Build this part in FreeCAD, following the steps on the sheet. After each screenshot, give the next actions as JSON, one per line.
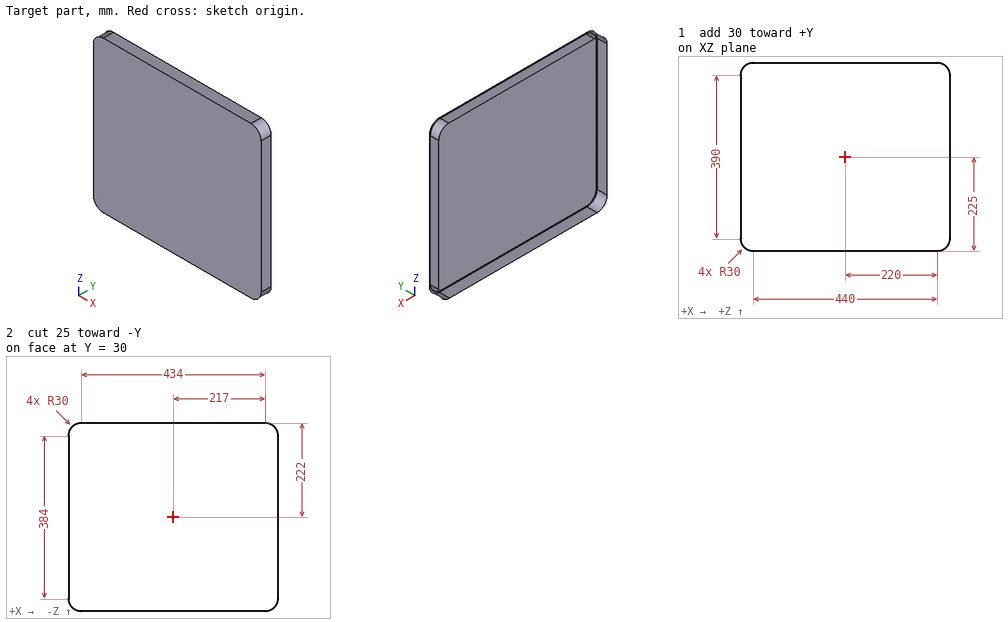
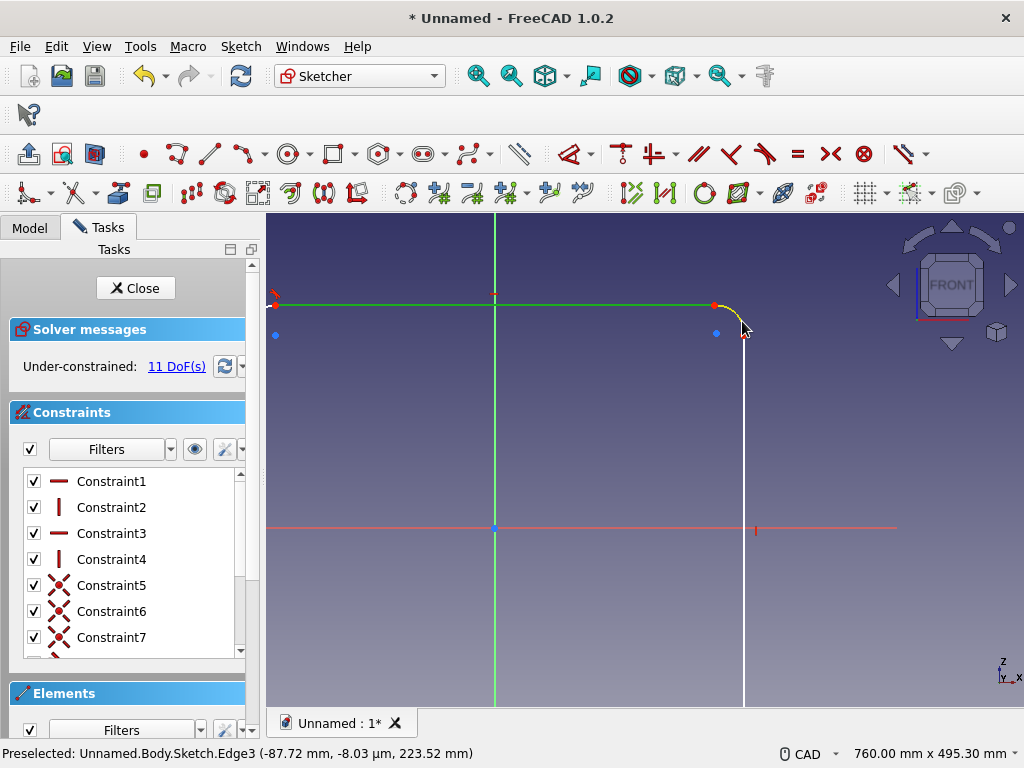
{"action": "left_click", "coordinate": [741, 321]}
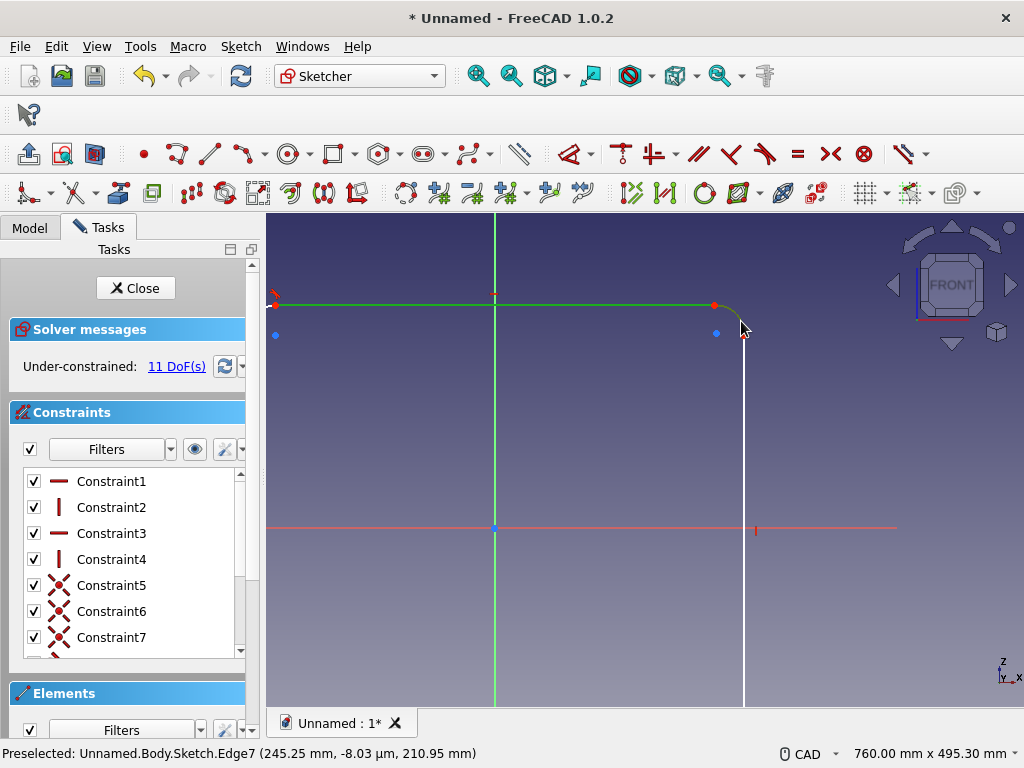
{"action": "left_click", "coordinate": [765, 154]}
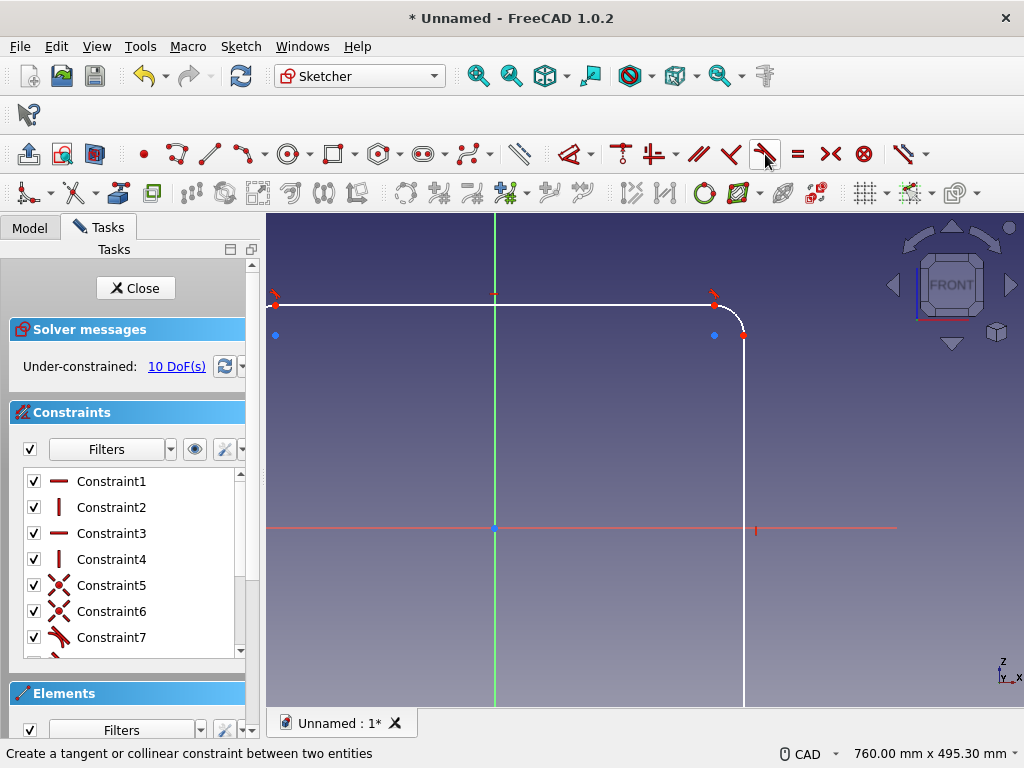
{"action": "left_click", "coordinate": [744, 452]}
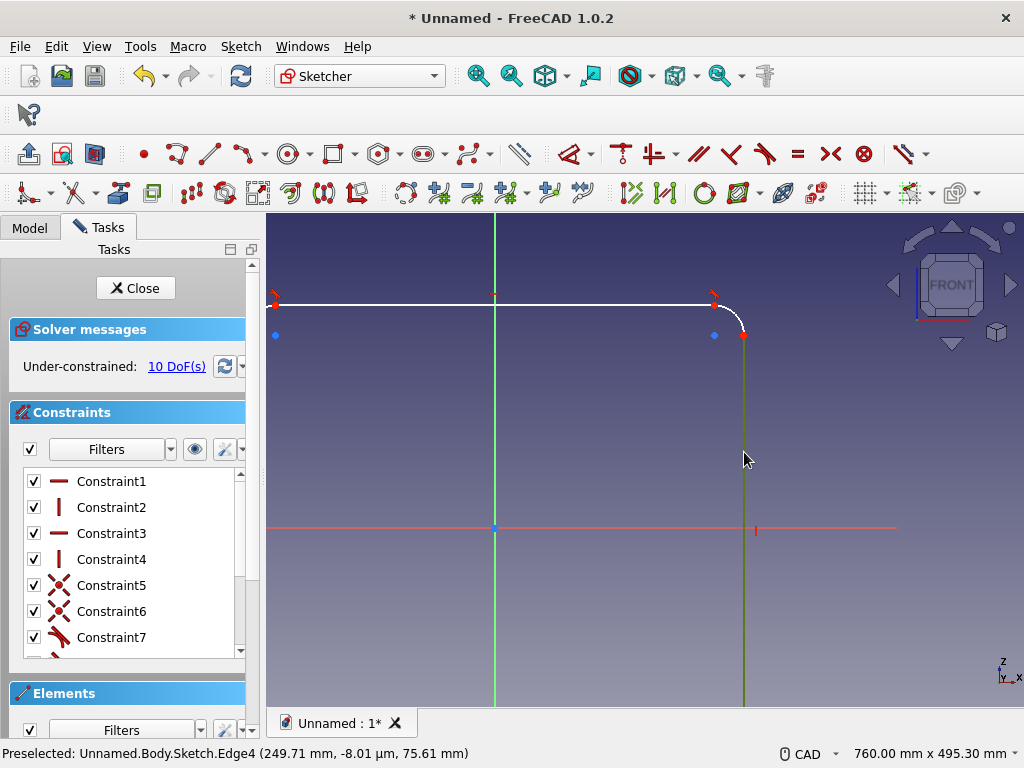
{"action": "left_click", "coordinate": [741, 322]}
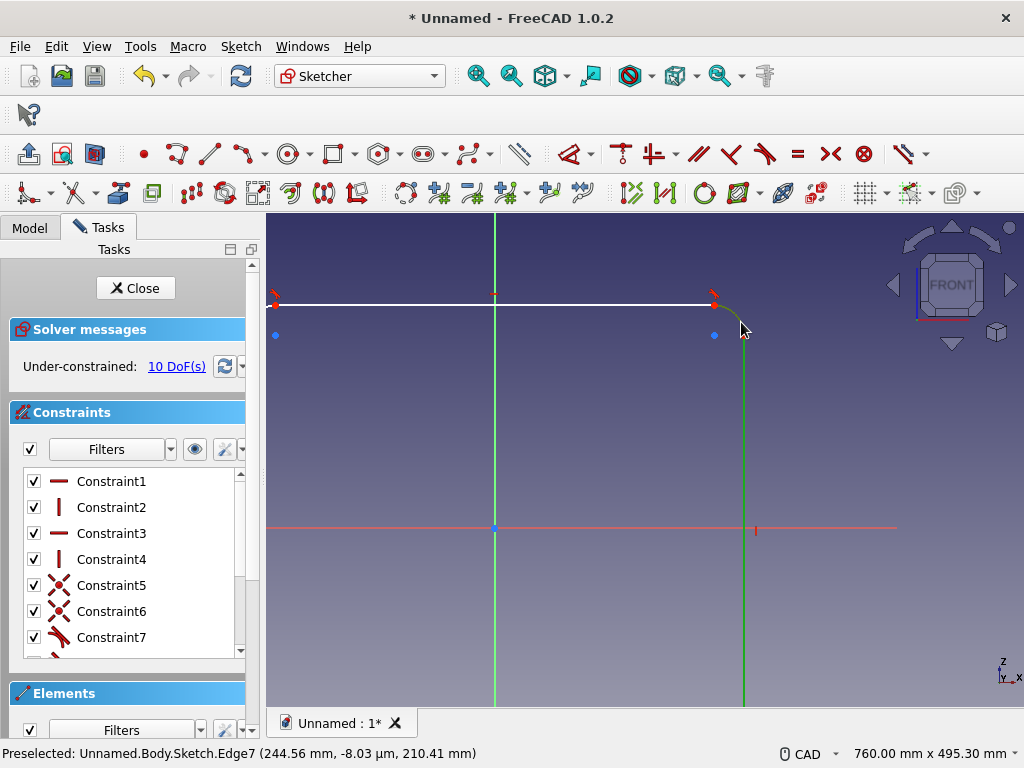
{"action": "left_click", "coordinate": [765, 154]}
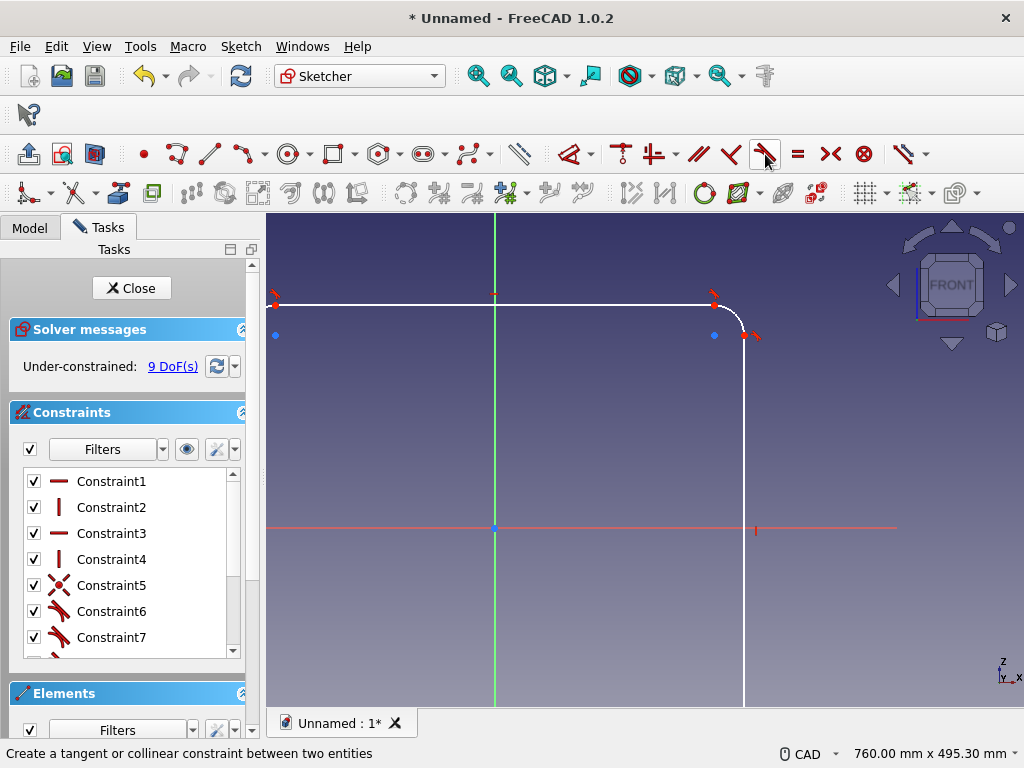
{"action": "left_click", "coordinate": [744, 452]}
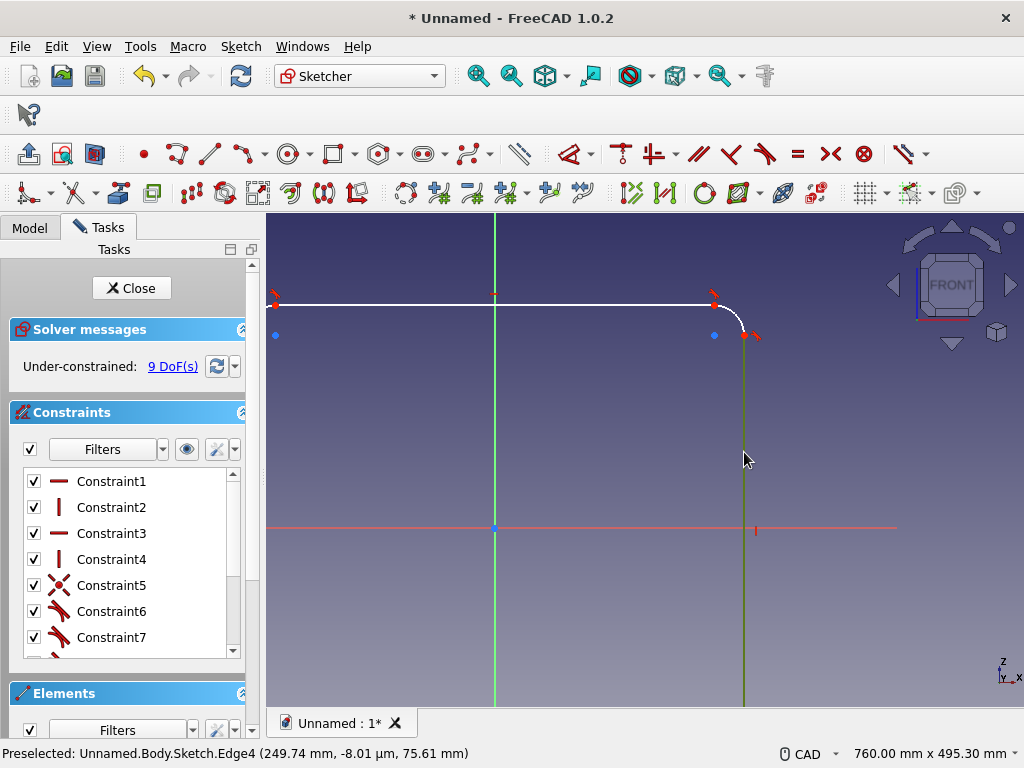
{"action": "scroll", "coordinate": [742, 321], "scroll_direction": "down", "scroll_amount": 2}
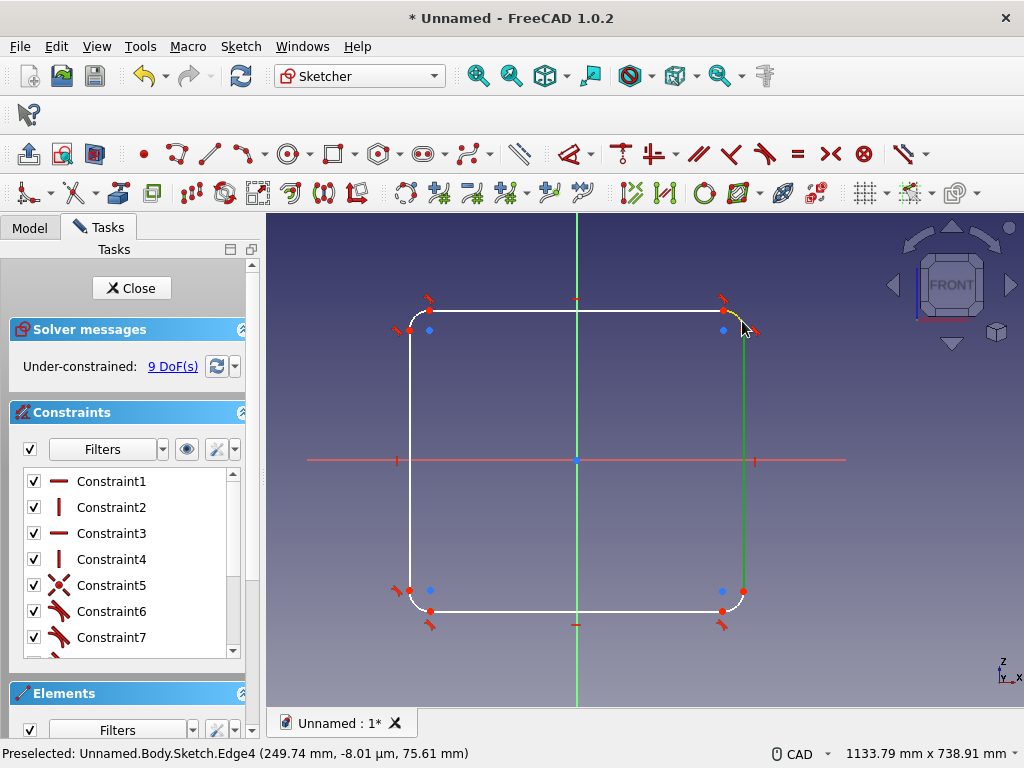
{"action": "scroll", "coordinate": [732, 610], "scroll_direction": "up", "scroll_amount": 2}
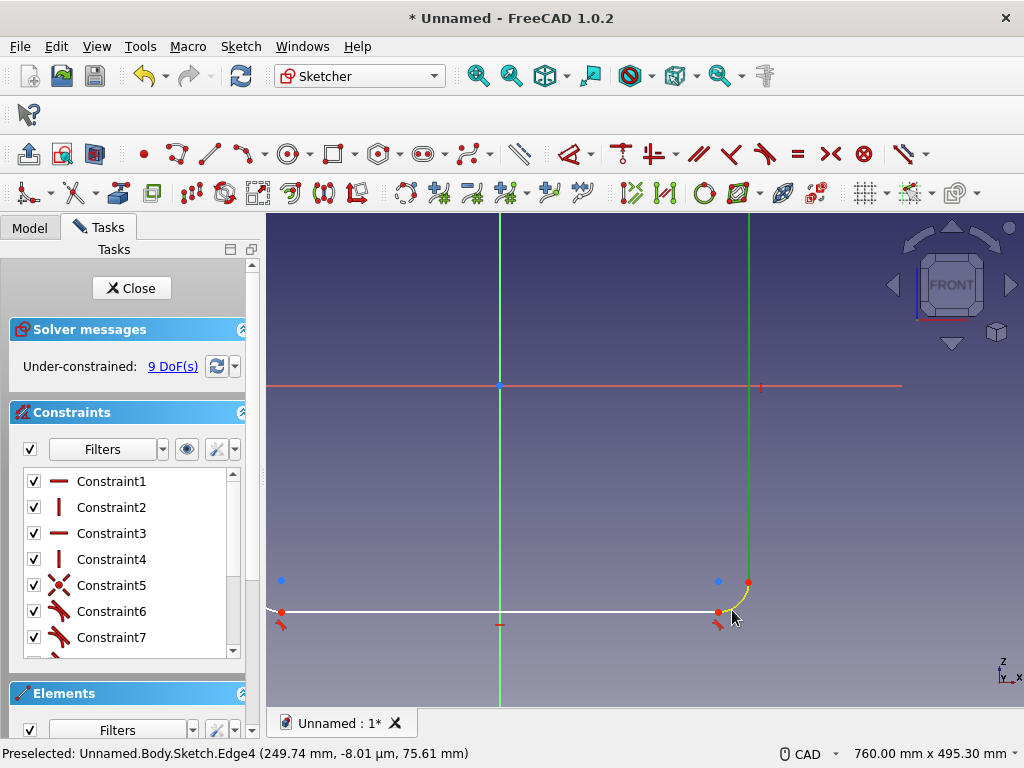
{"action": "left_click", "coordinate": [732, 609]}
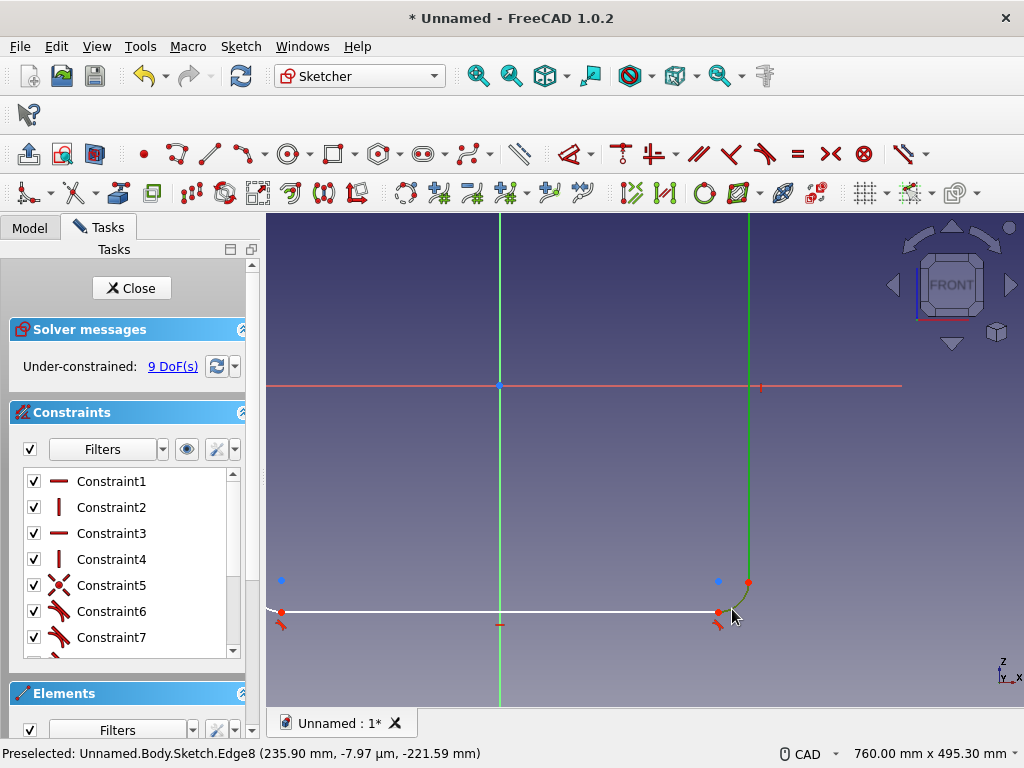
{"action": "left_click", "coordinate": [765, 154]}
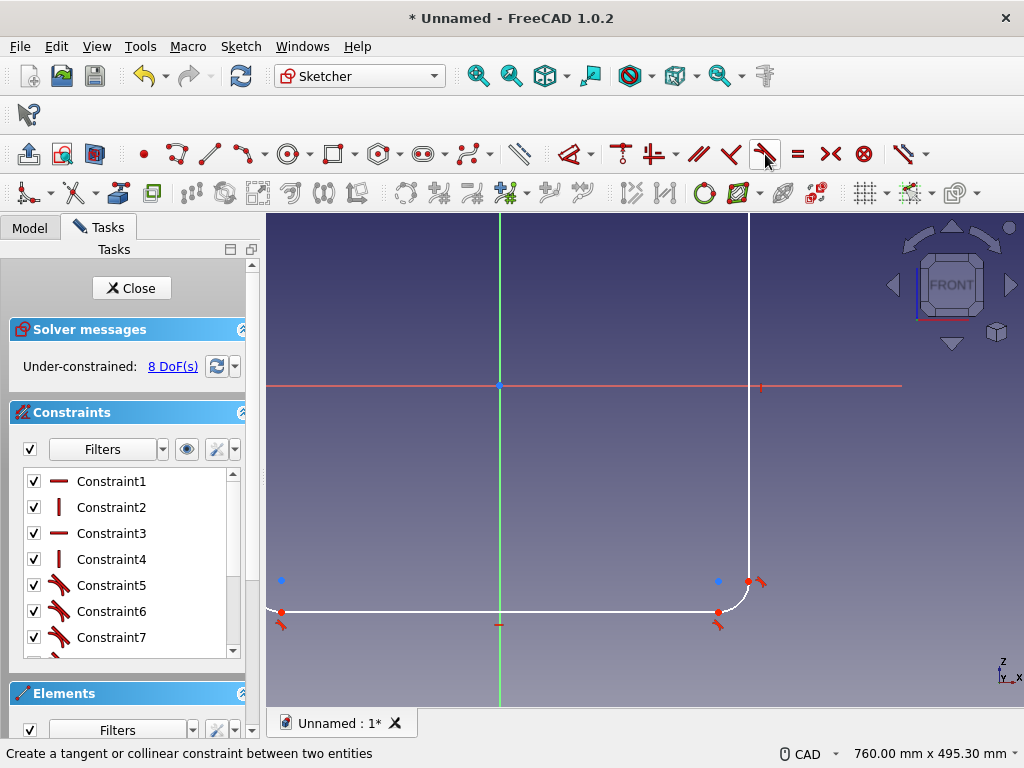
{"action": "scroll", "coordinate": [732, 610], "scroll_direction": "down", "scroll_amount": 2}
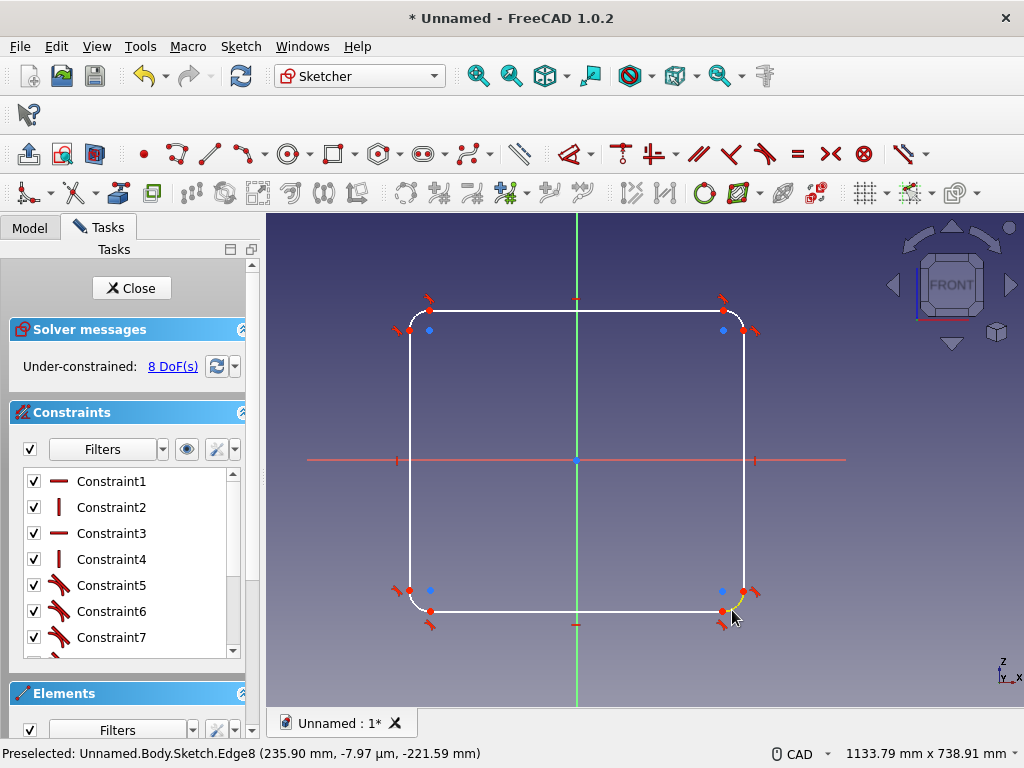
{"action": "scroll", "coordinate": [412, 600], "scroll_direction": "up", "scroll_amount": 2}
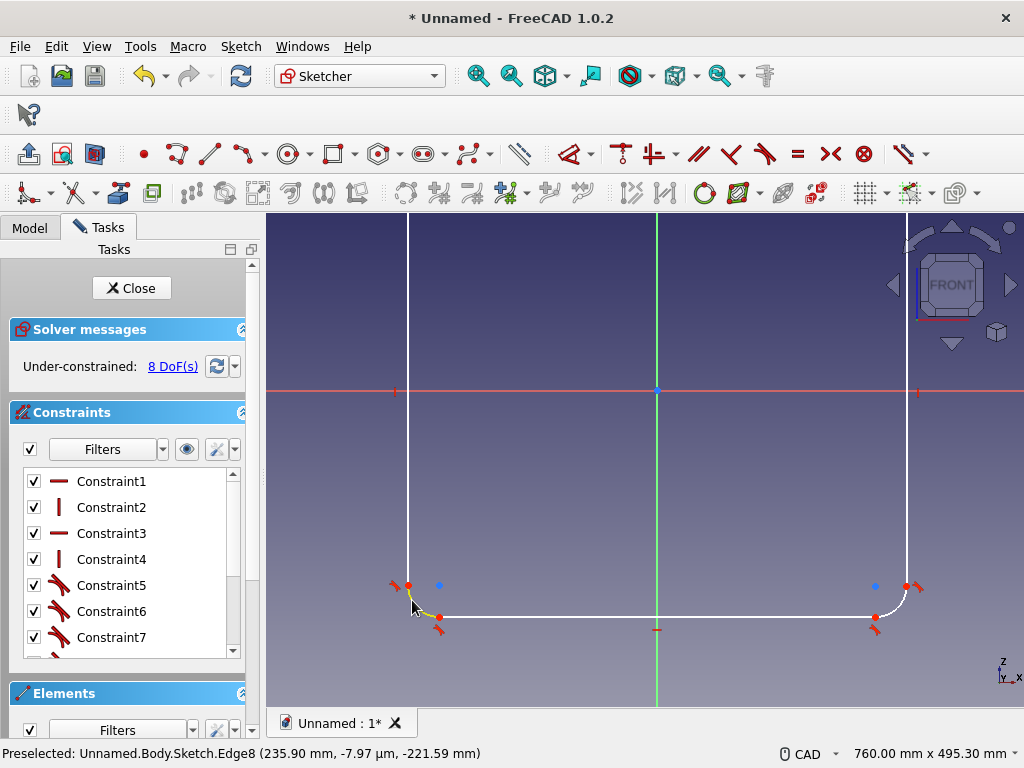
{"action": "left_click", "coordinate": [412, 600]}